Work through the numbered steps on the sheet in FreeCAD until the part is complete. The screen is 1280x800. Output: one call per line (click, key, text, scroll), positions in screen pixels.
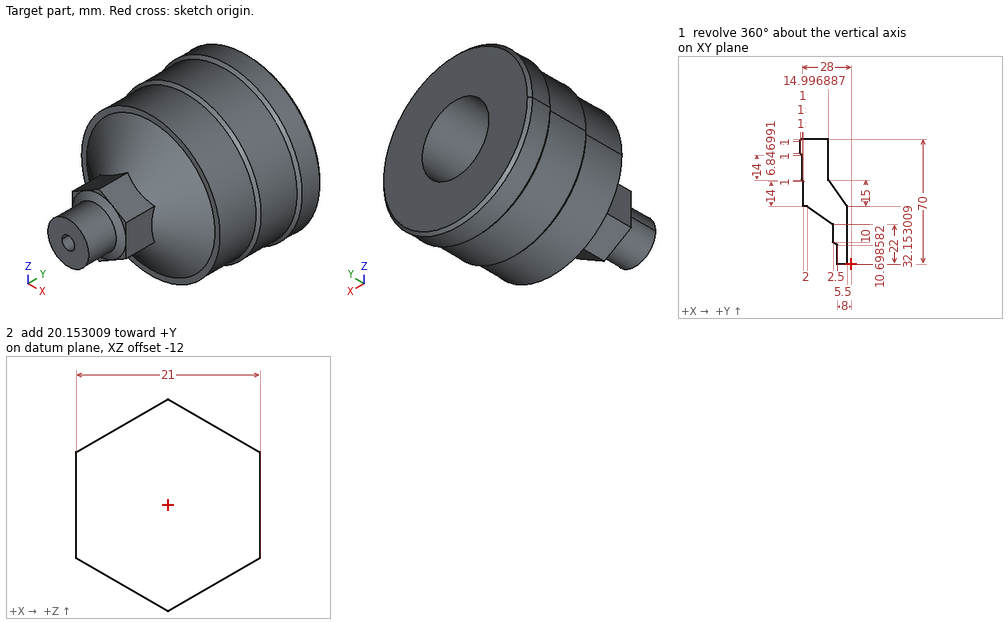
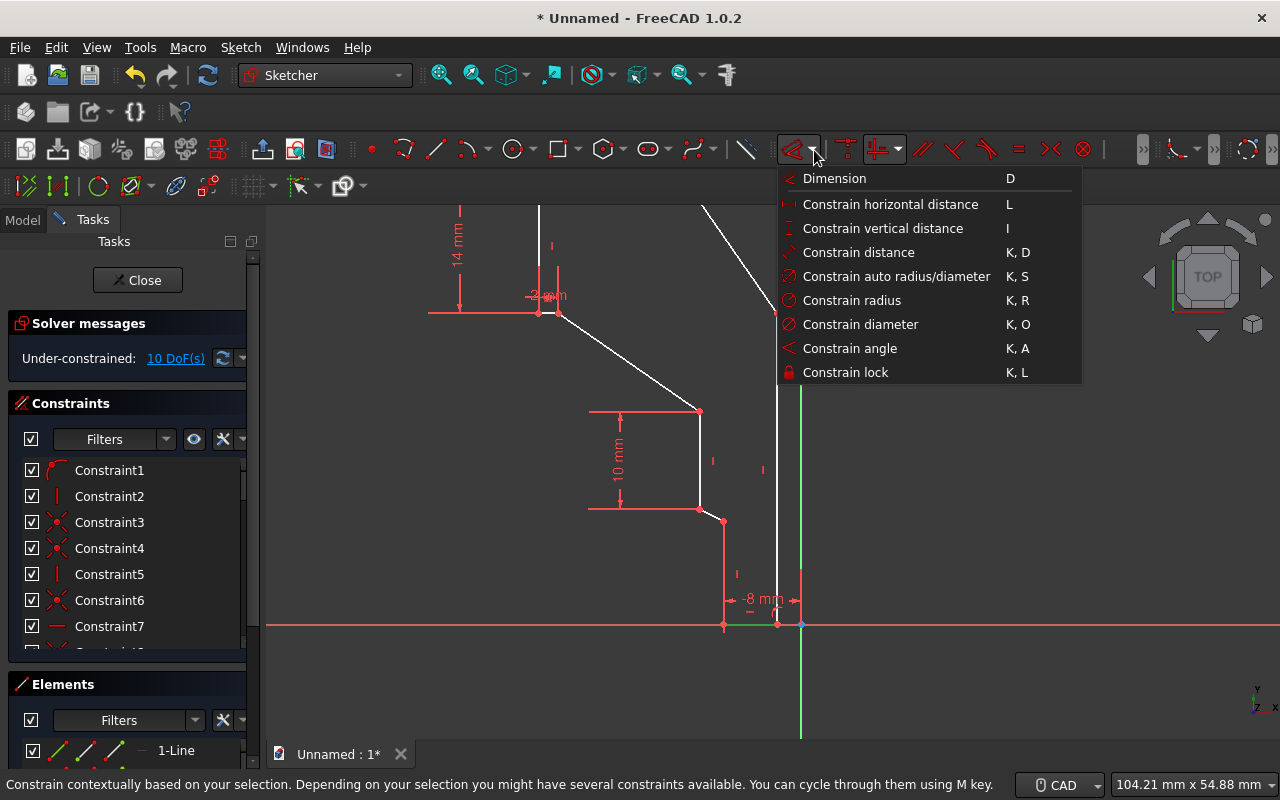
click(930, 204)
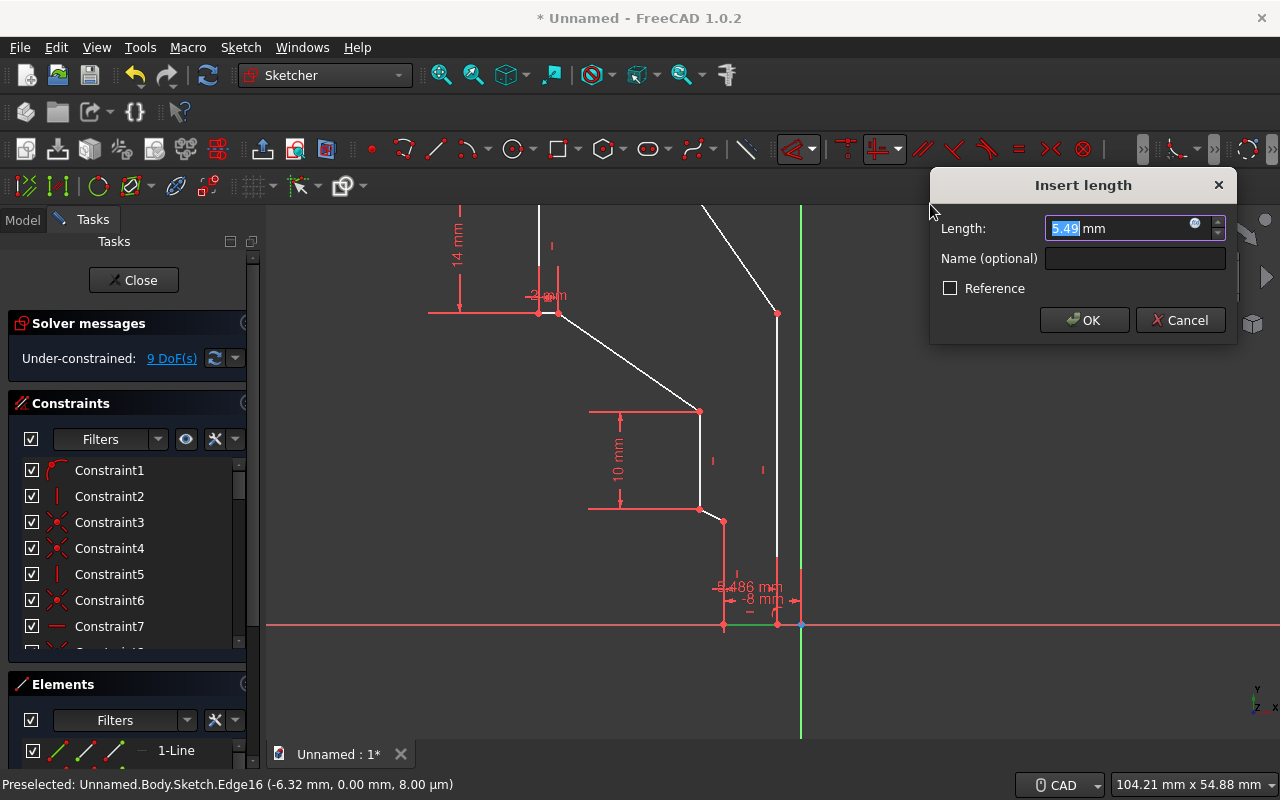
text(5.5)
key(Return)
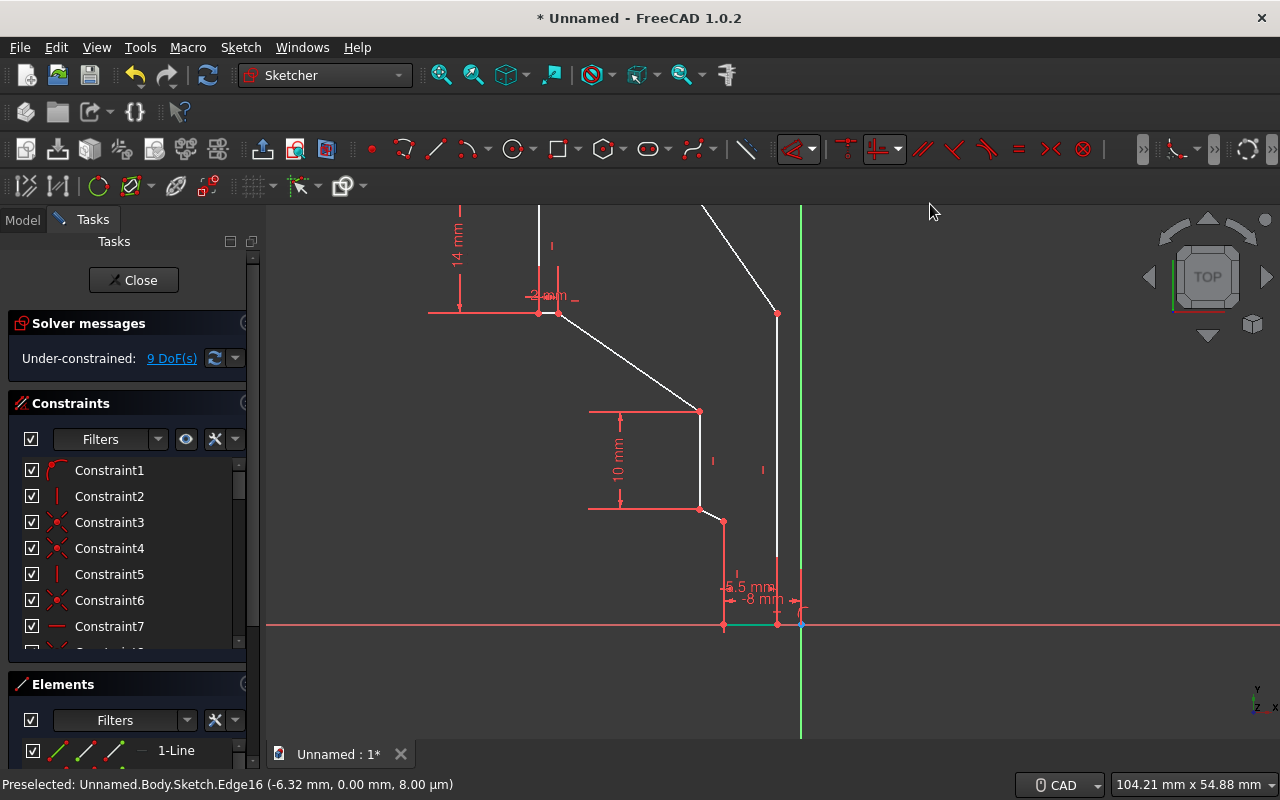
scroll(740, 625, down, 4)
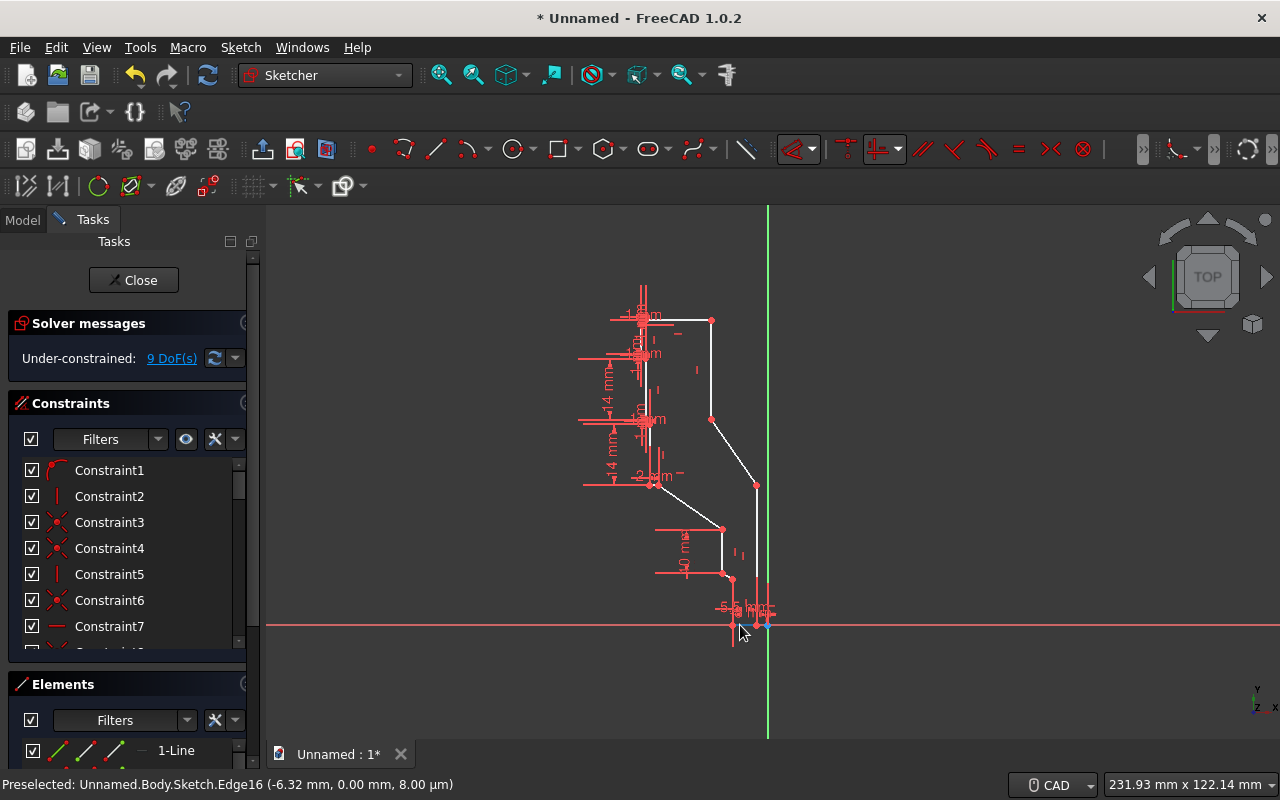
click(711, 320)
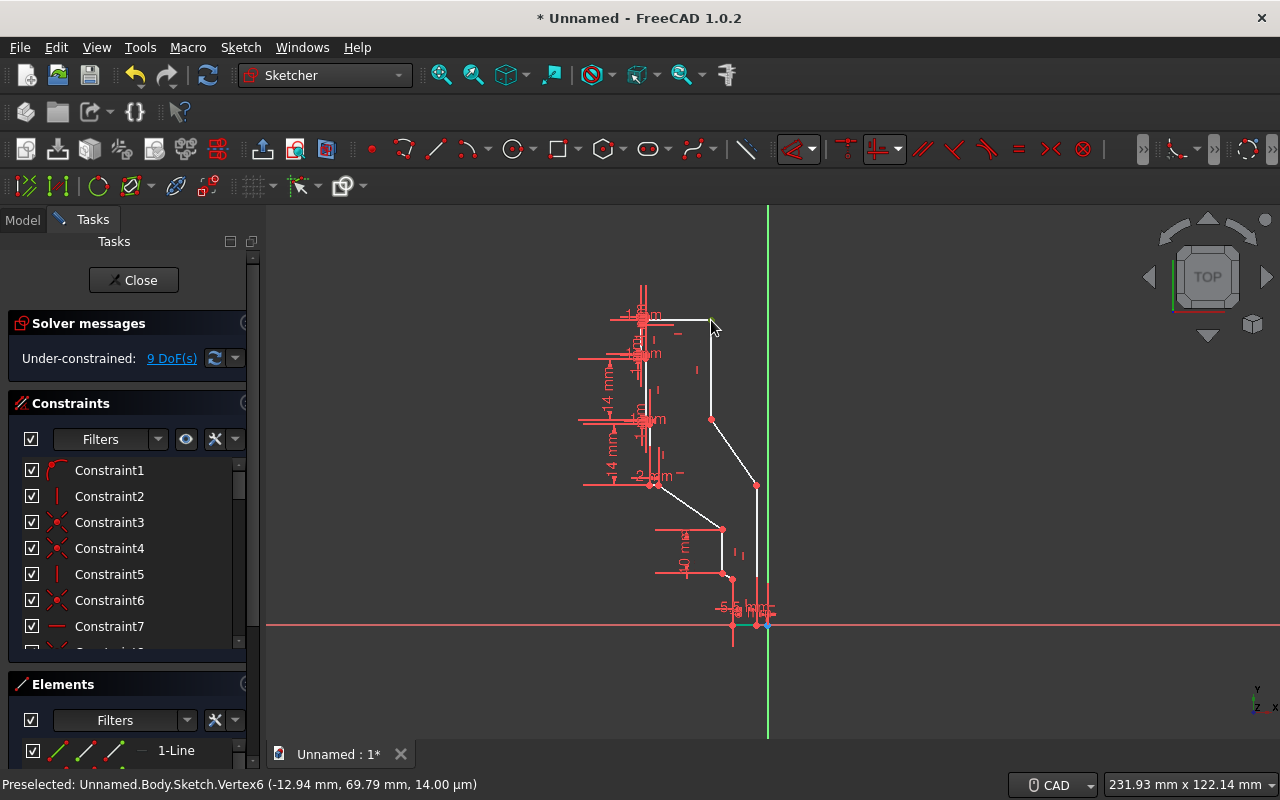
key(i)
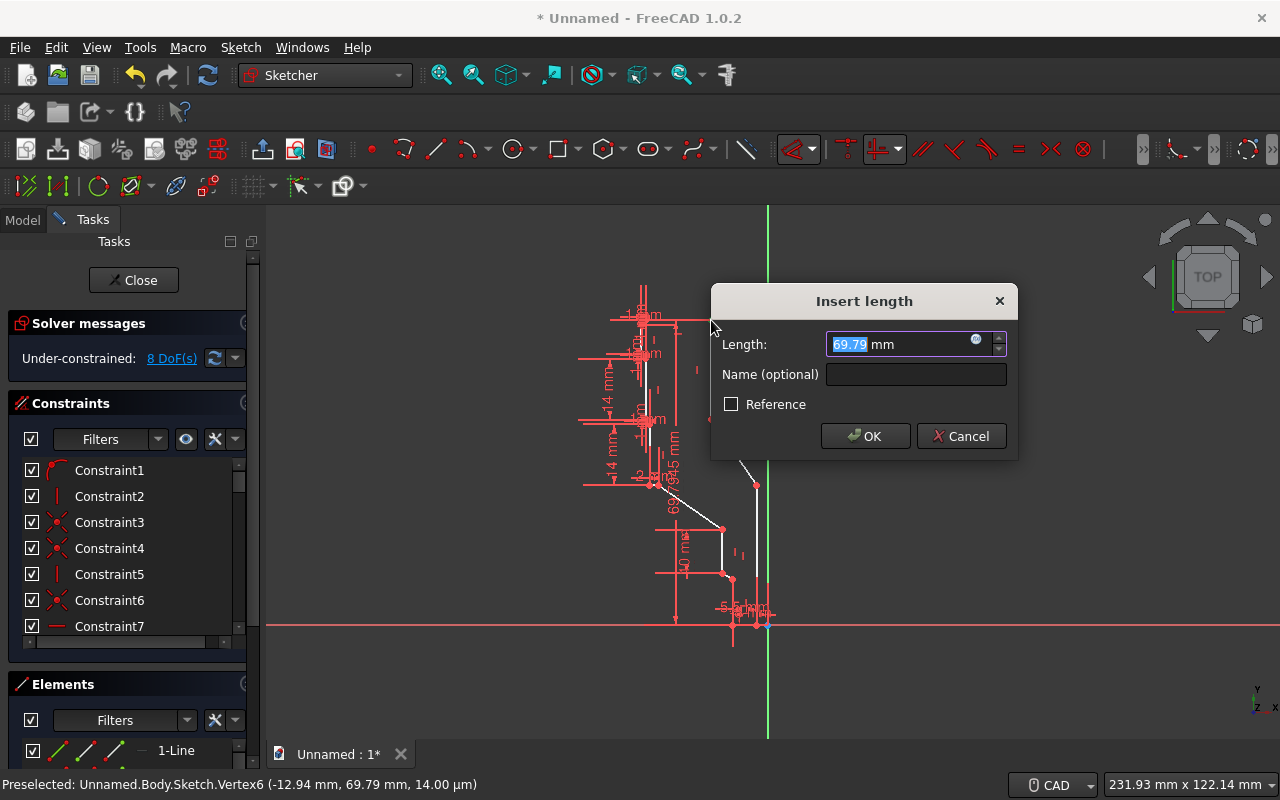
text(70)
key(Return)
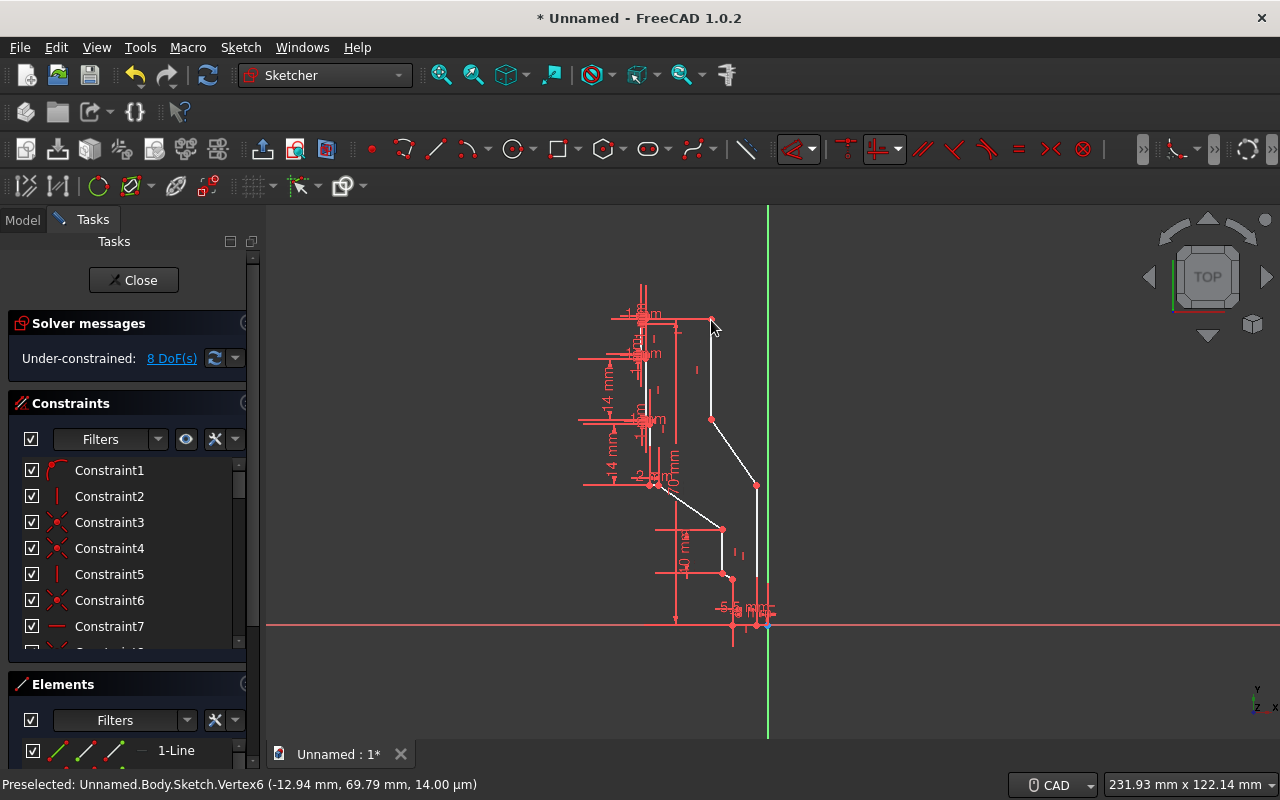
scroll(646, 319, up, 4)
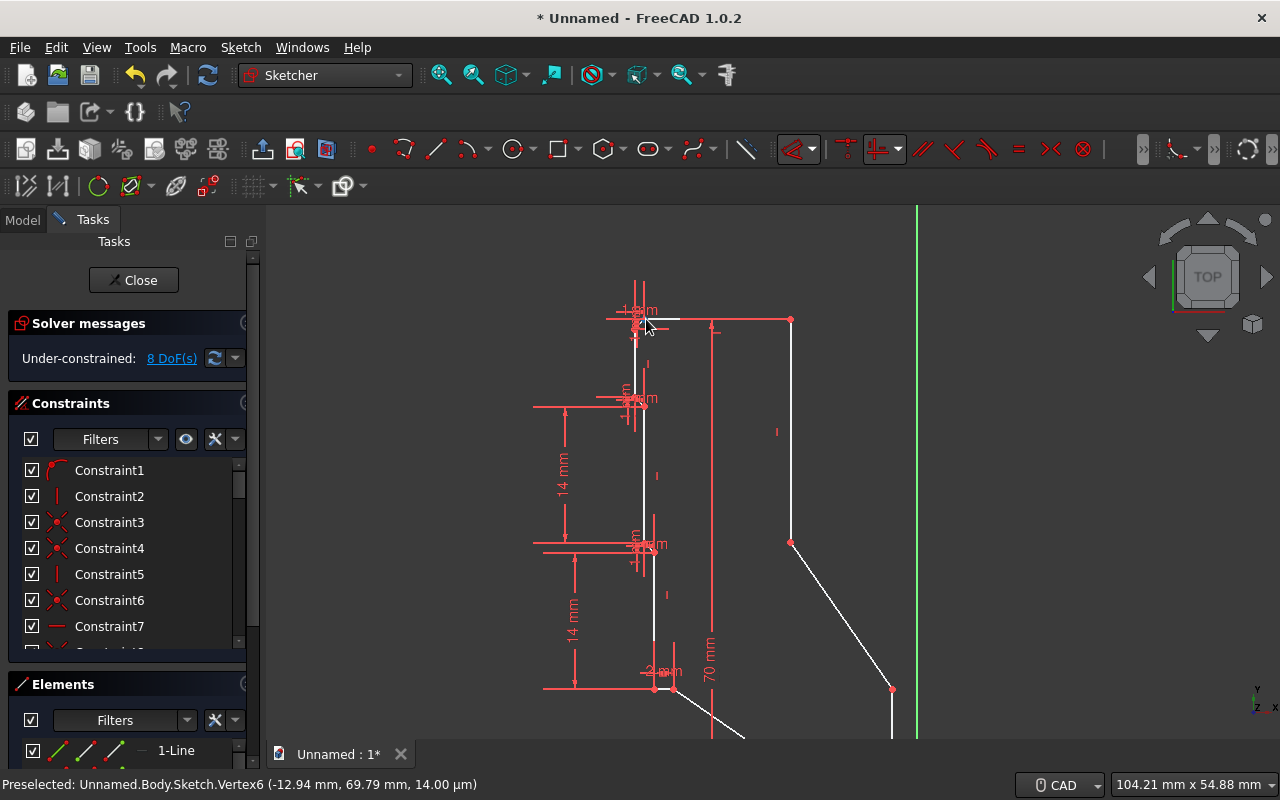
click(644, 319)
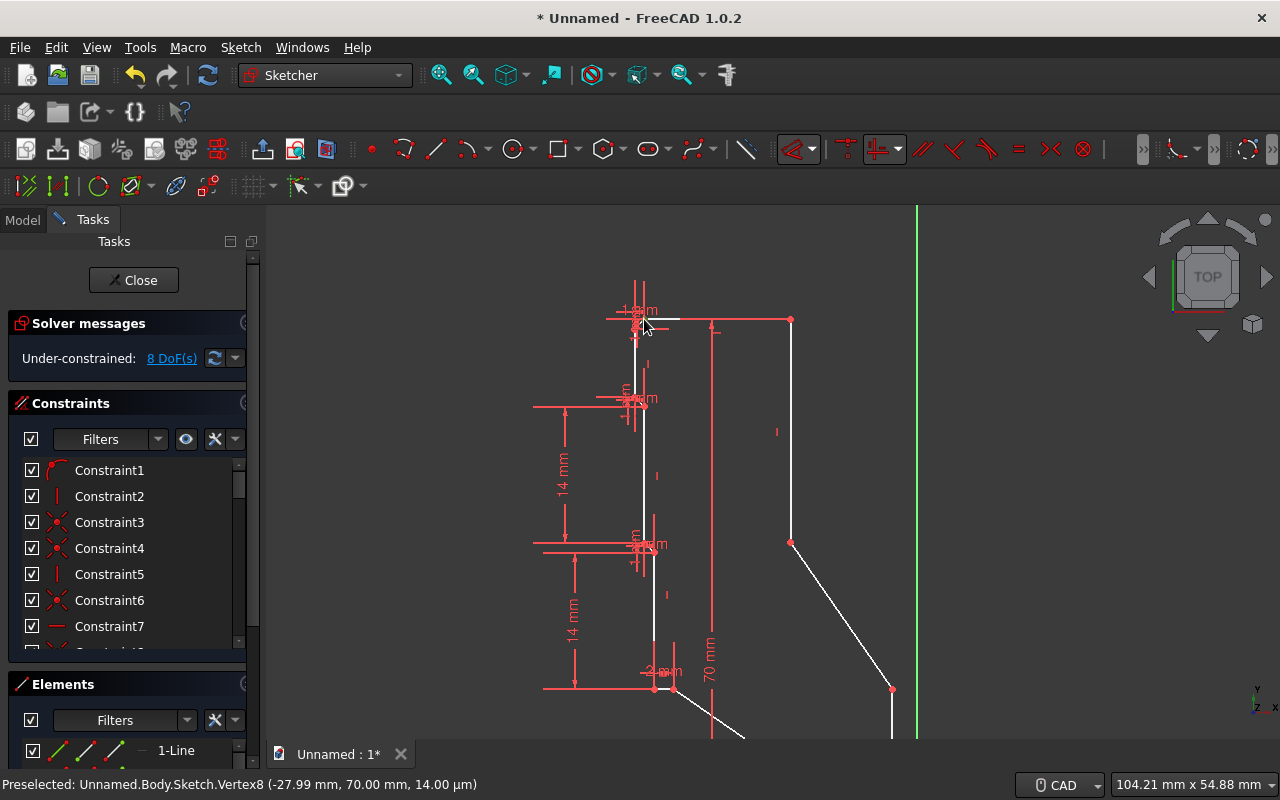
key(l)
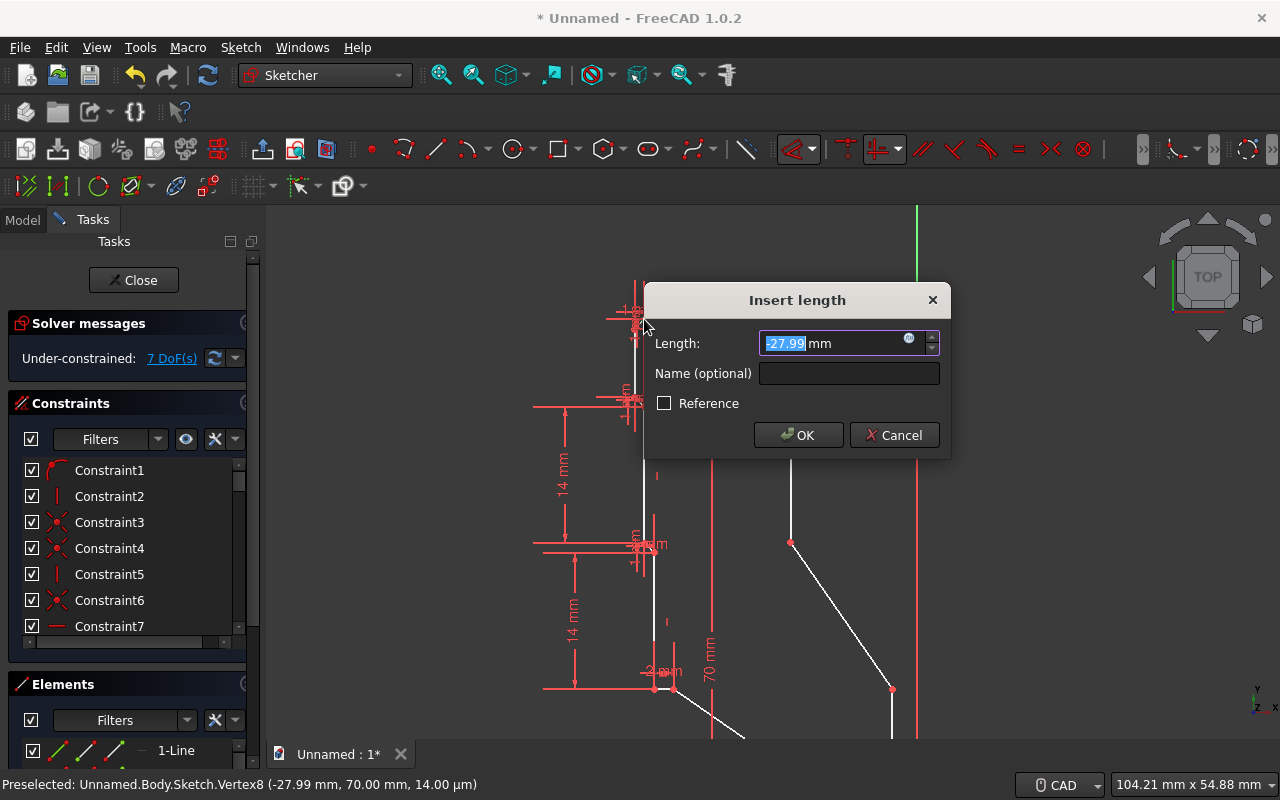
text(-28)
key(Return)